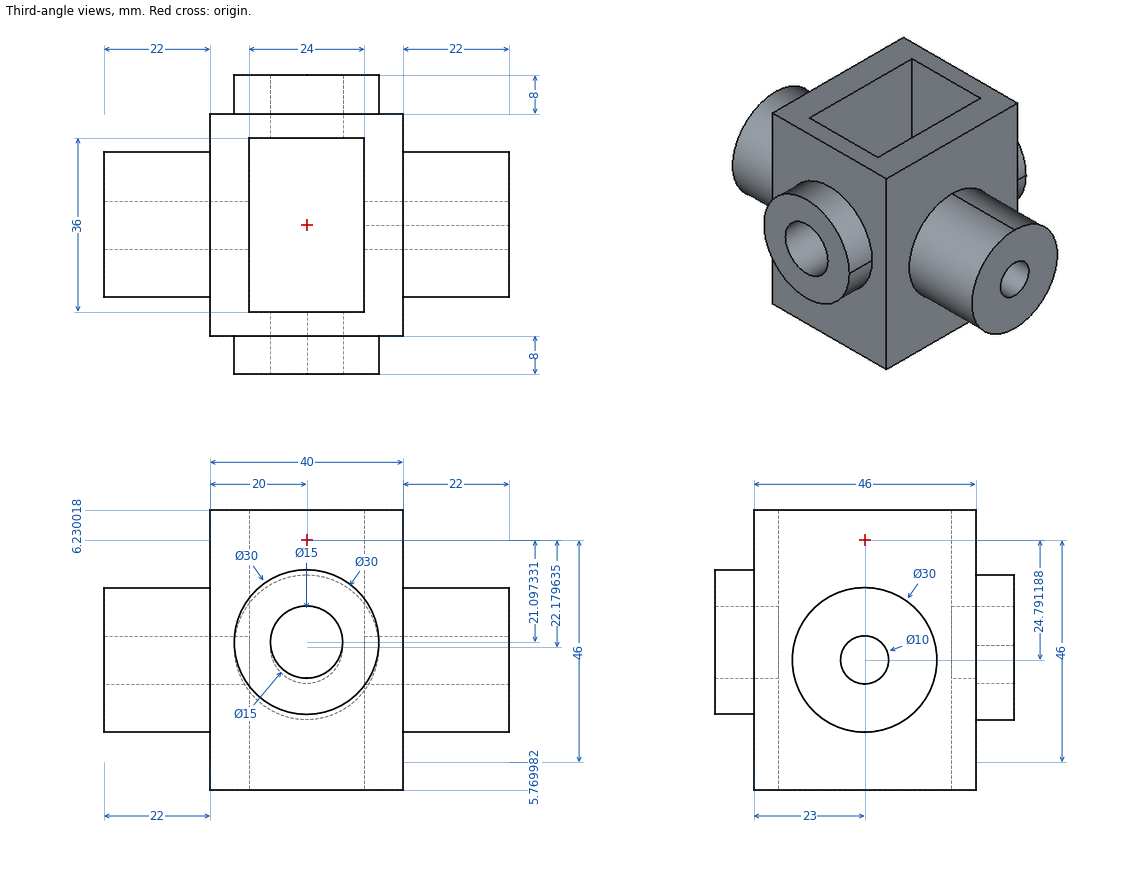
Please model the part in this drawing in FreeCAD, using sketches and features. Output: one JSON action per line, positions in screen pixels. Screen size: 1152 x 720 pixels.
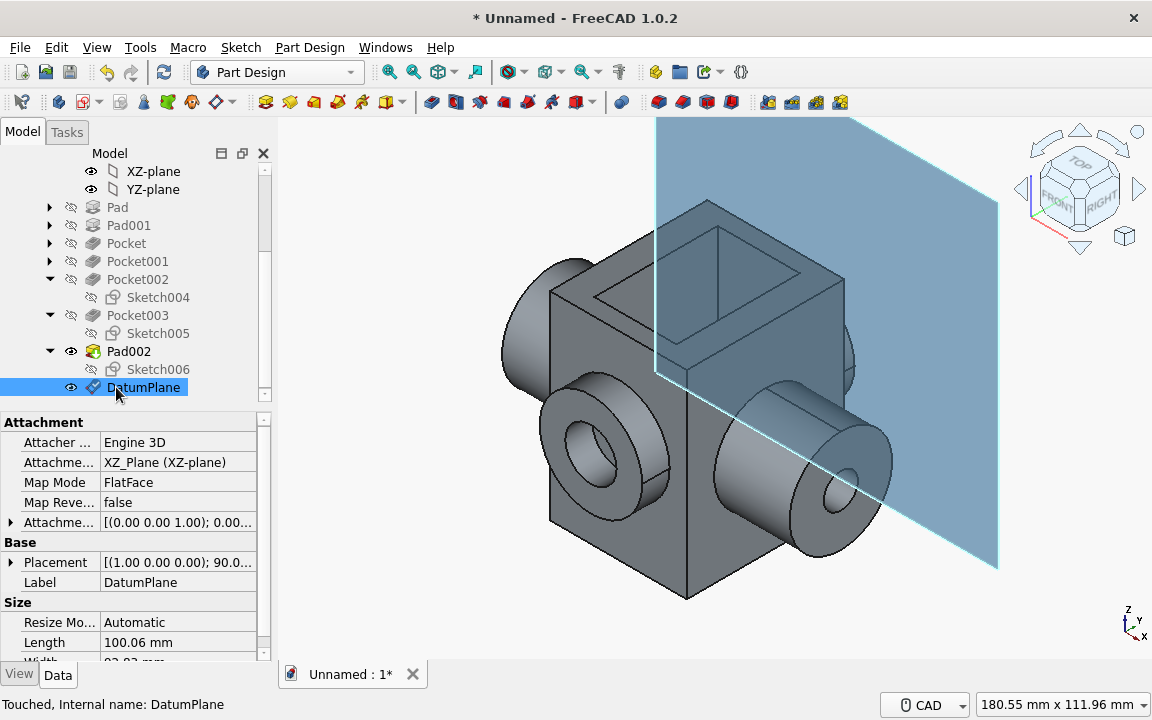
{"action": "left_click", "coordinate": [84, 102]}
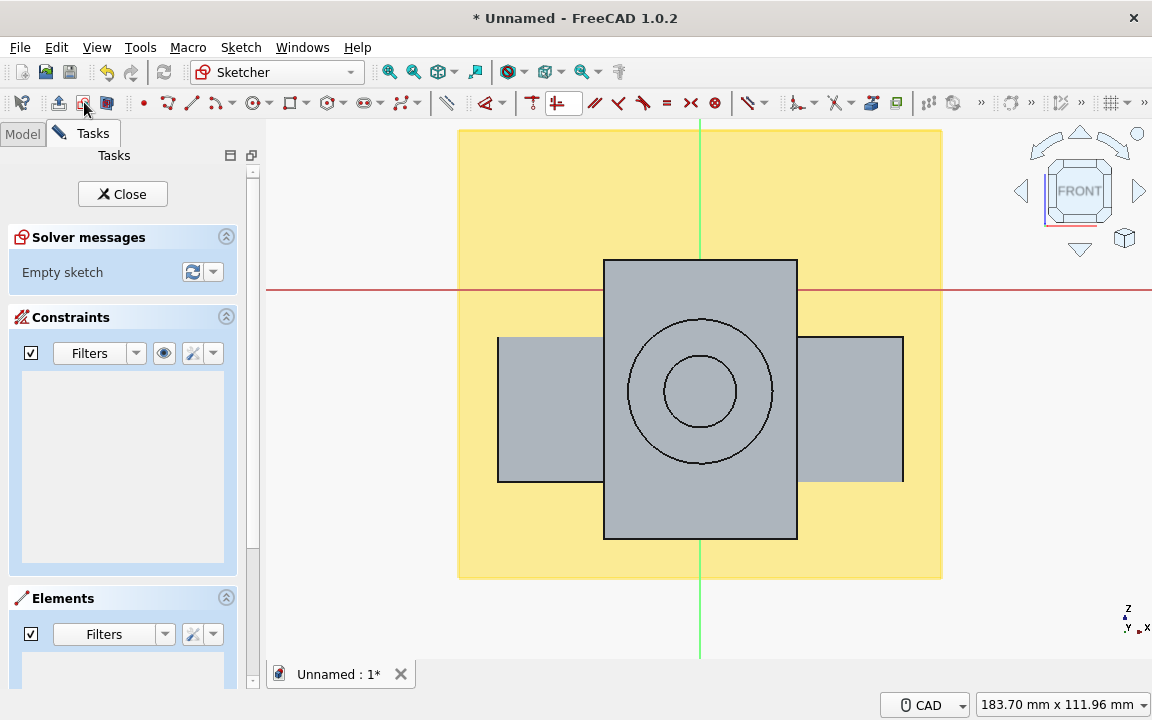
{"action": "left_click", "coordinate": [108, 104]}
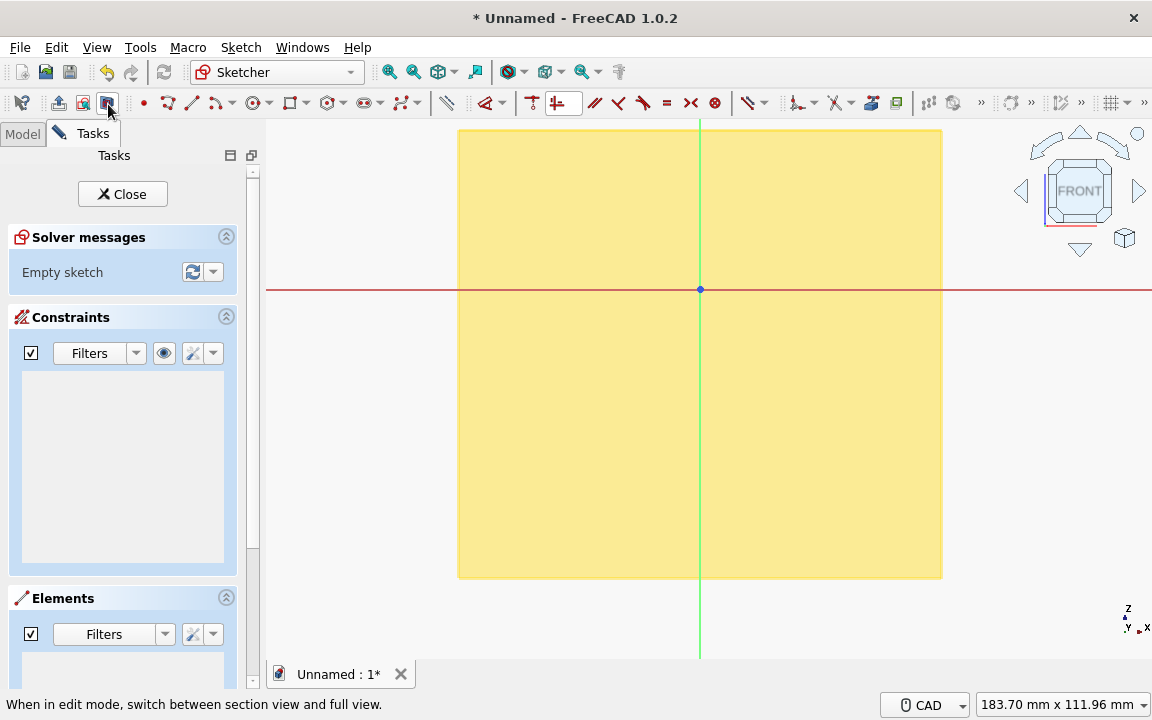
{"action": "scroll", "coordinate": [735, 341], "scroll_direction": "up", "scroll_amount": 5}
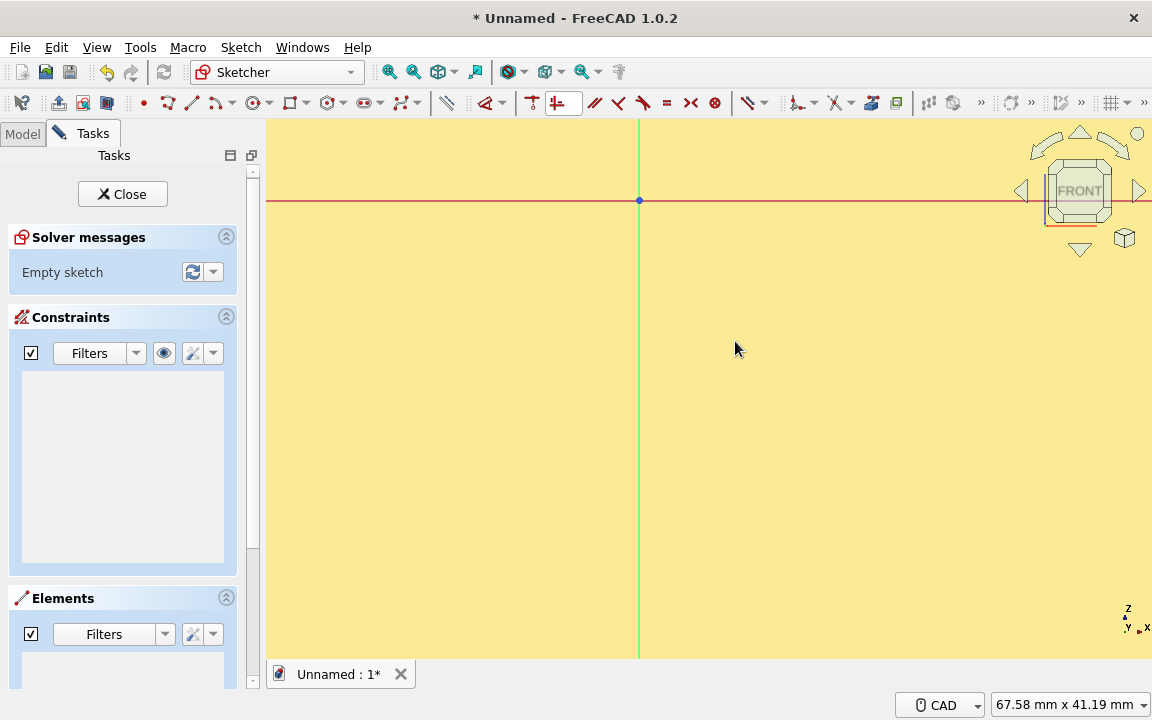
{"action": "left_click", "coordinate": [254, 104]}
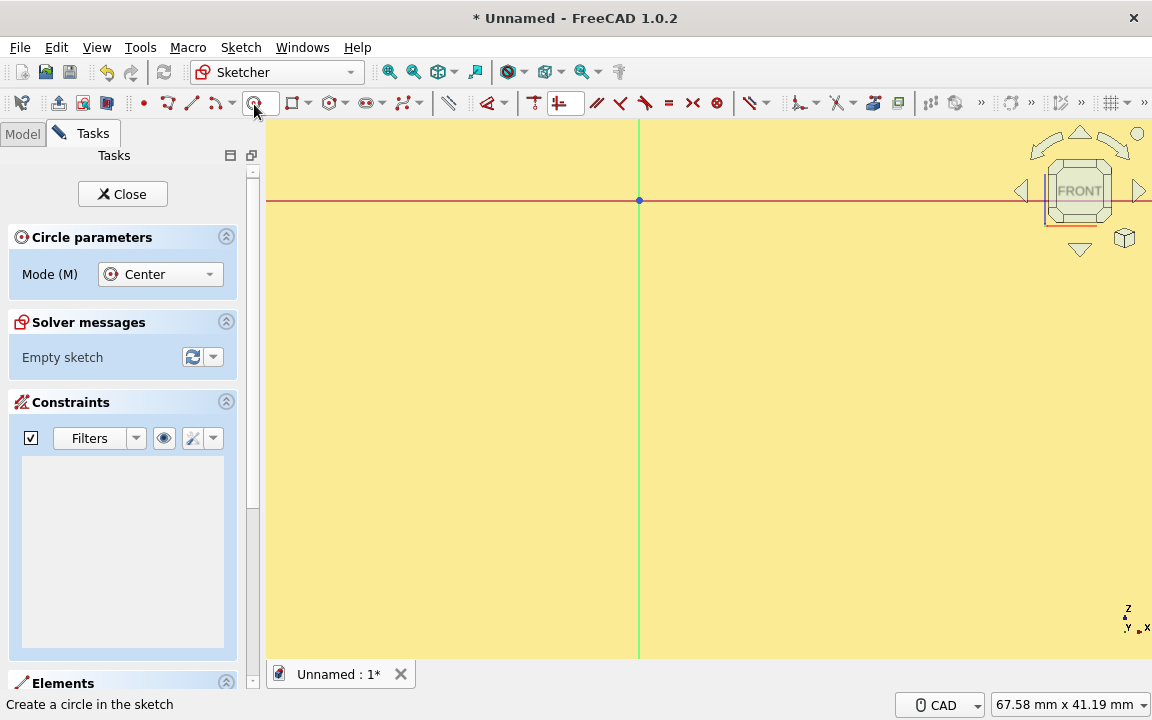
{"action": "left_click", "coordinate": [639, 478]}
{"action": "left_click", "coordinate": [709, 408]}
{"action": "key", "text": "Escape"}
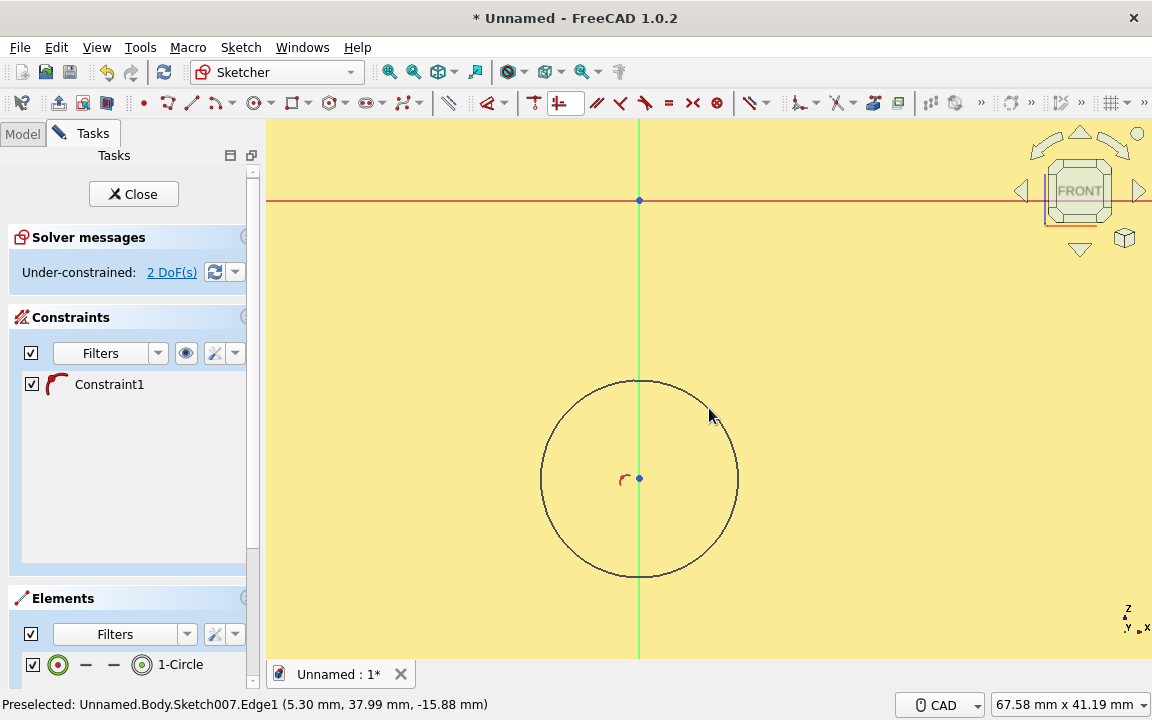
{"action": "left_click", "coordinate": [488, 104]}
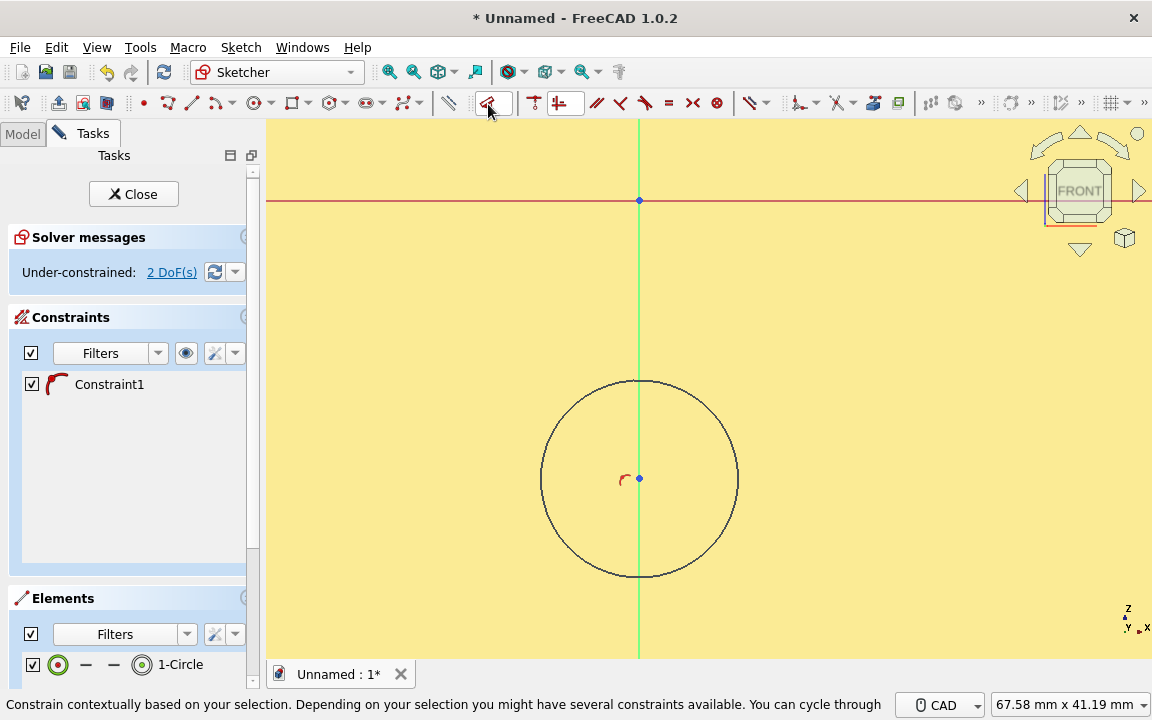
{"action": "left_click", "coordinate": [709, 409]}
{"action": "left_click", "coordinate": [732, 386]}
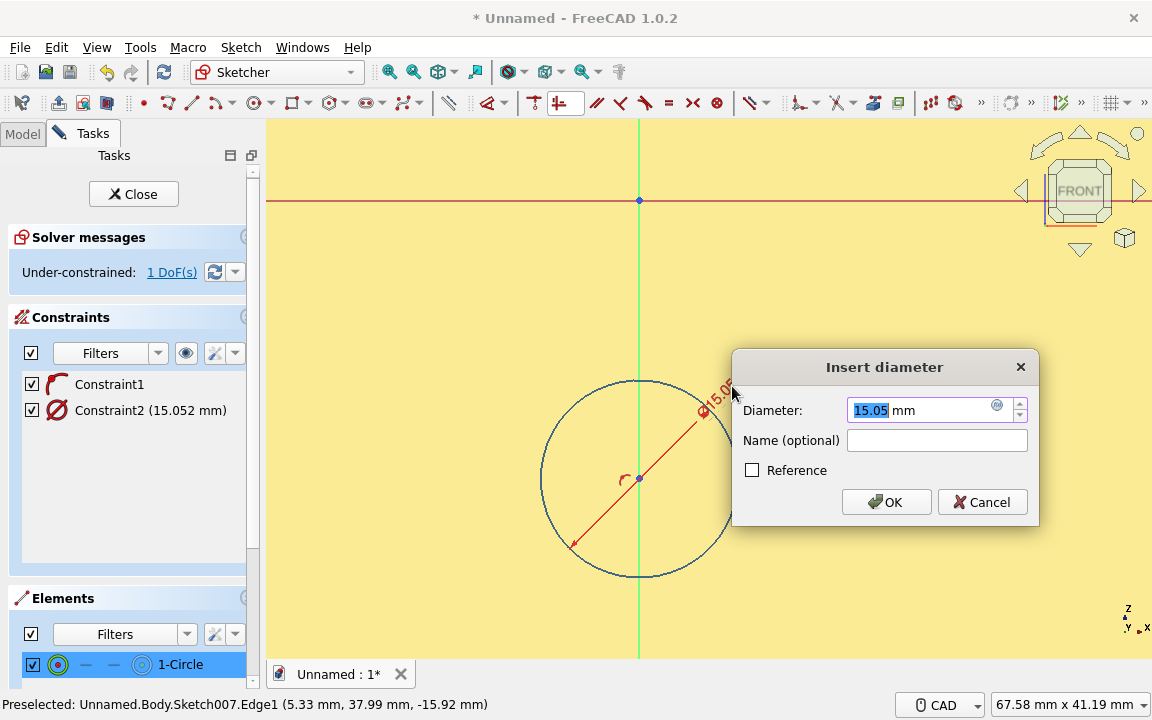
{"action": "type", "text": "15"}
{"action": "key", "text": "Return"}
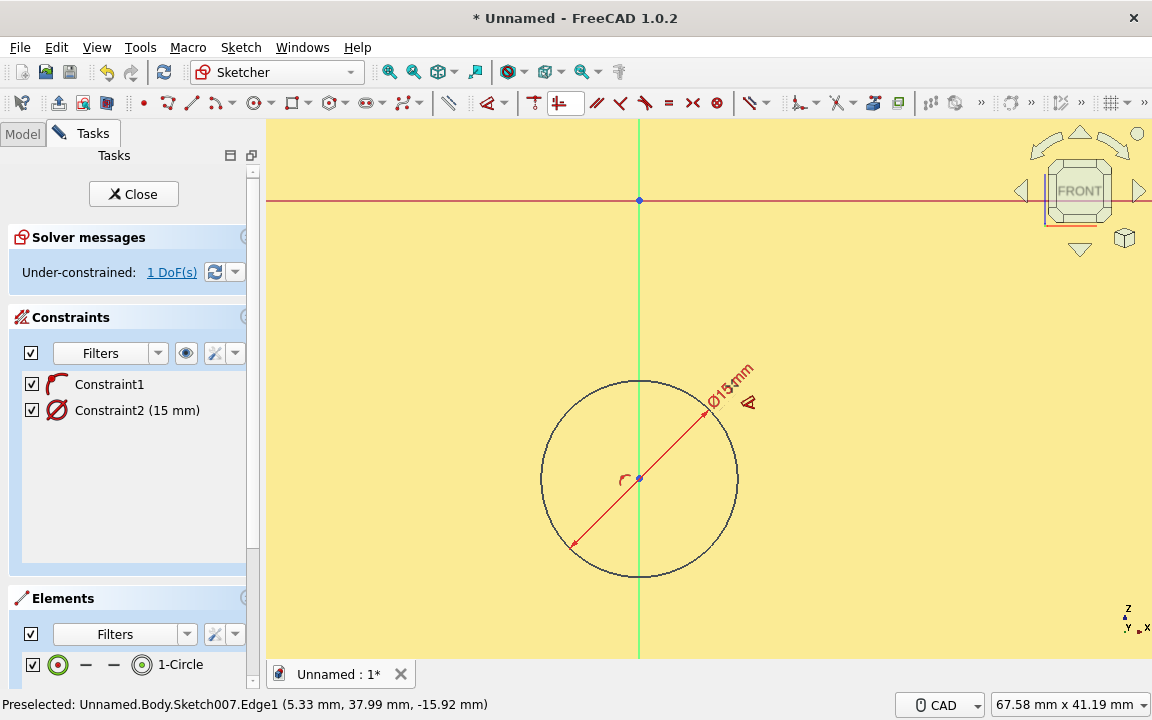
{"action": "left_click", "coordinate": [639, 479]}
{"action": "left_click", "coordinate": [673, 340]}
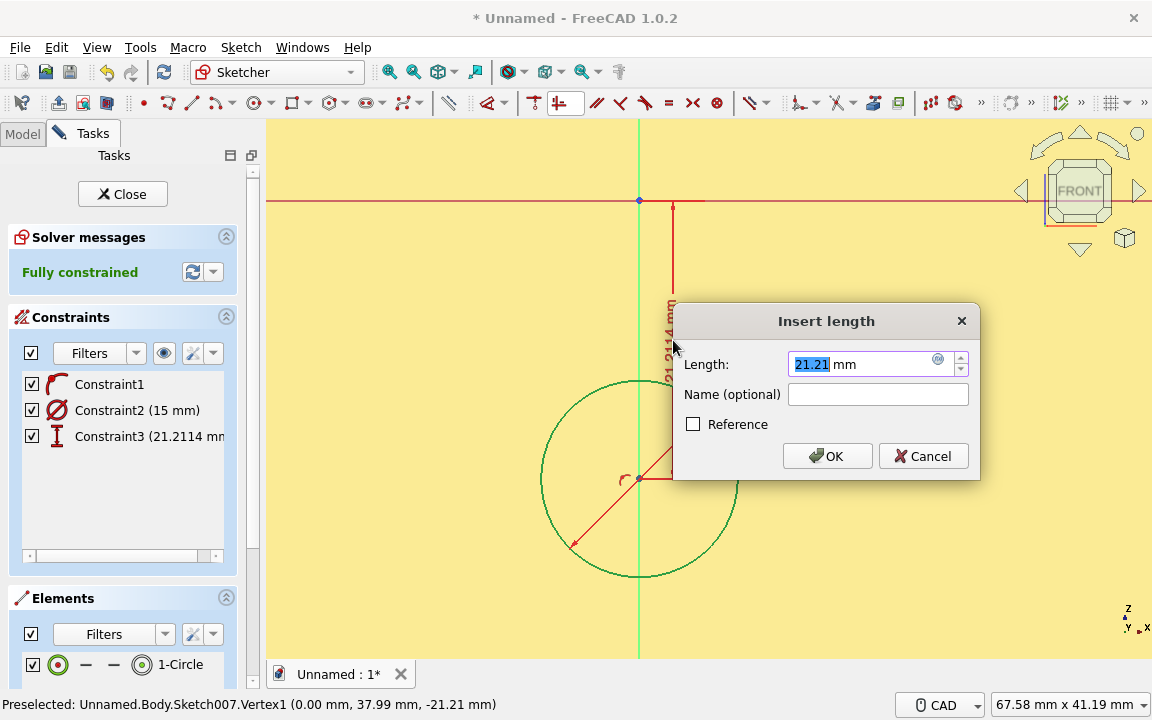
{"action": "type", "text": "21.097331"}
{"action": "key", "text": "Return"}
{"action": "key", "text": "Escape"}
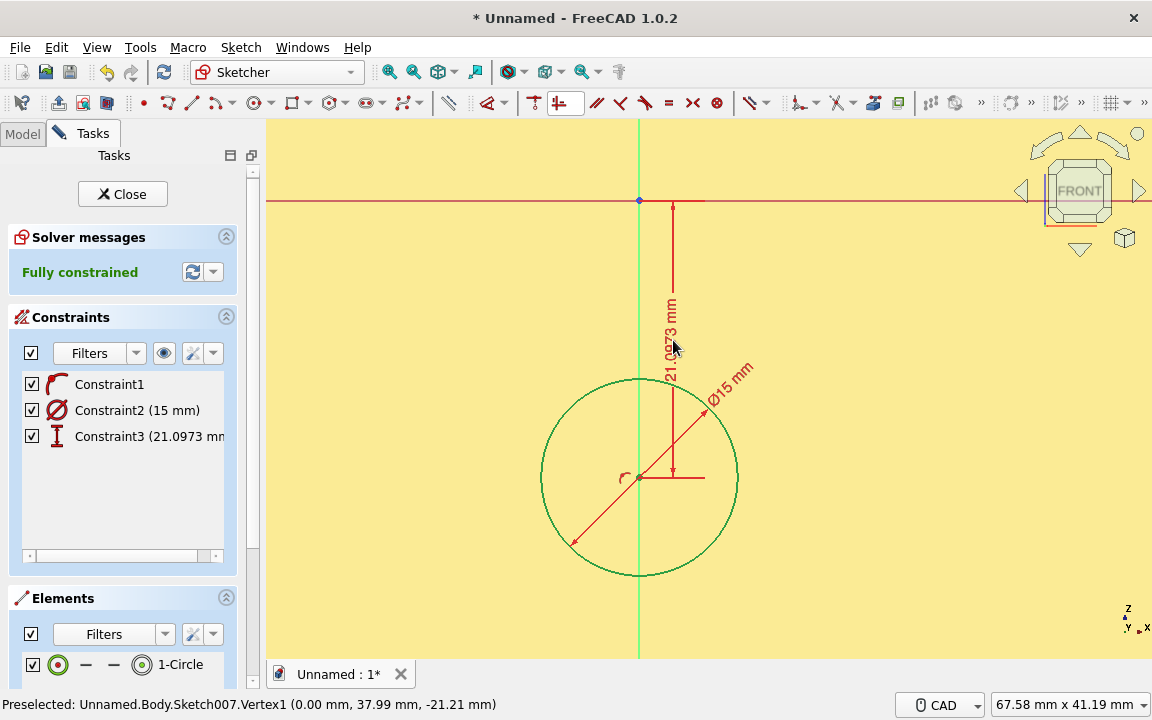
{"action": "left_click", "coordinate": [123, 194]}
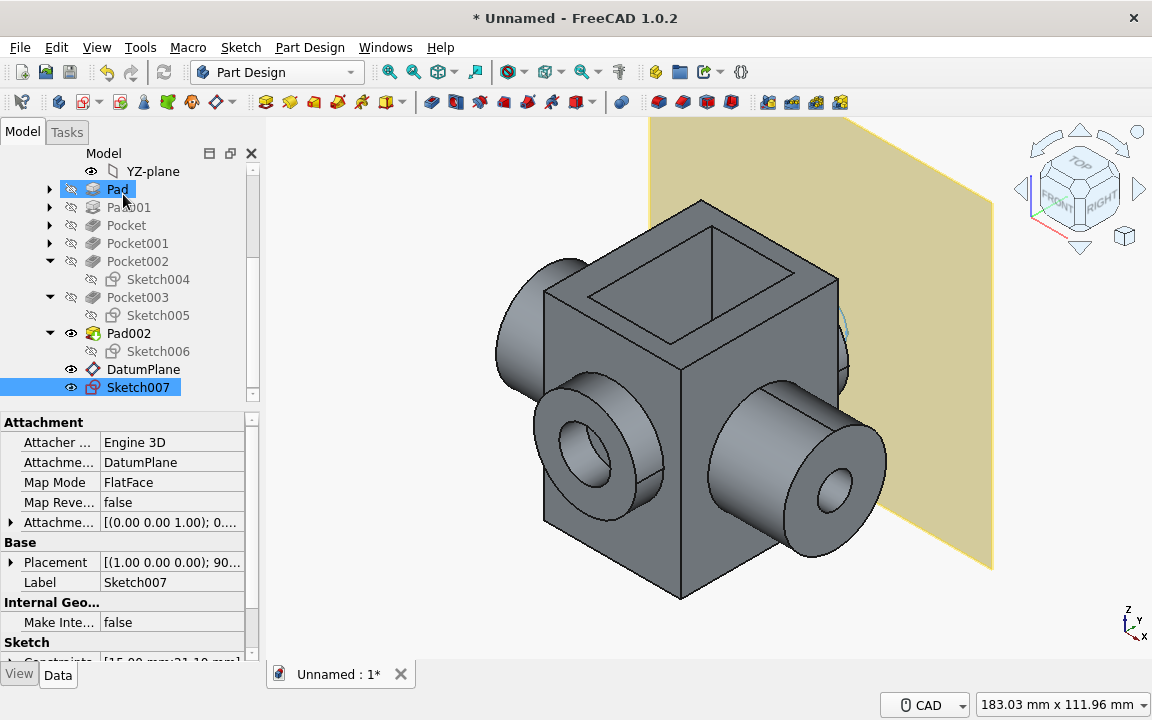
{"action": "left_click", "coordinate": [432, 102]}